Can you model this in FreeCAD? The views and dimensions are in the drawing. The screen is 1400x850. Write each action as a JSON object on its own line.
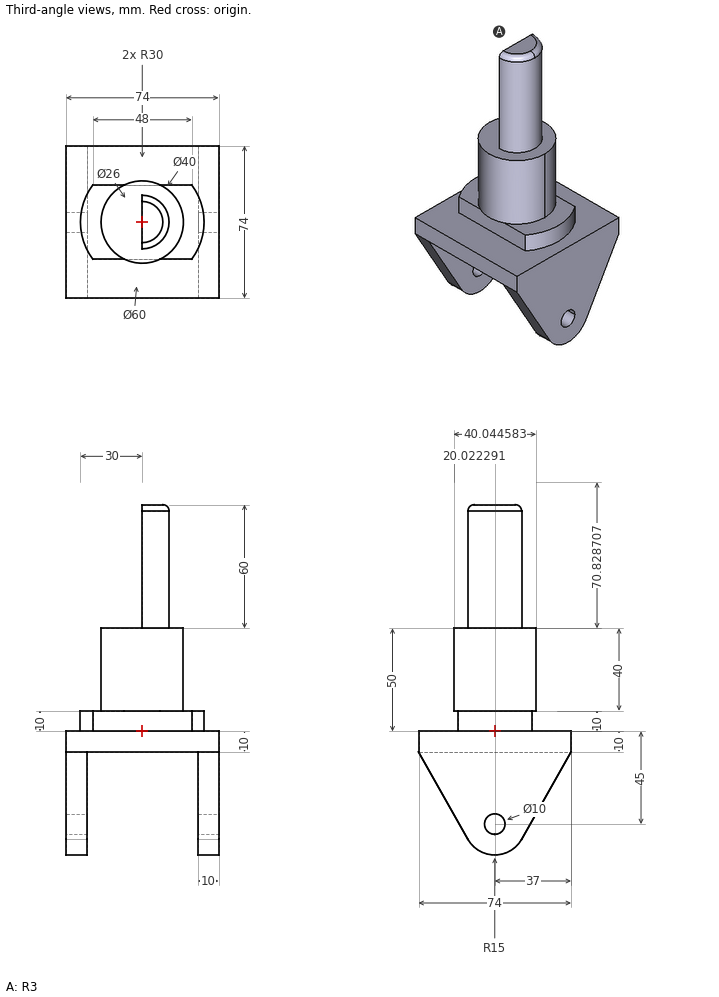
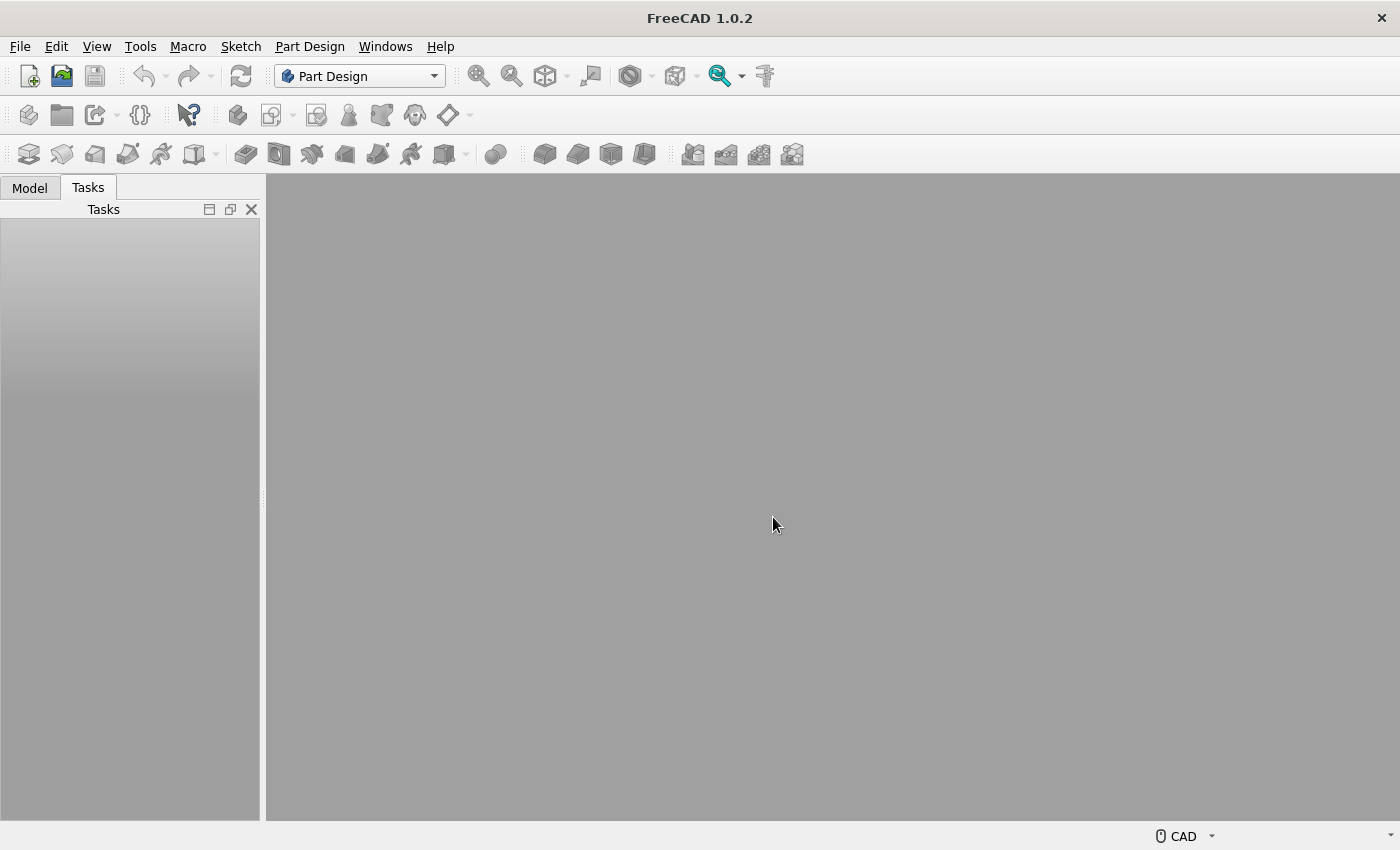
{"action": "key", "text": "ctrl+n"}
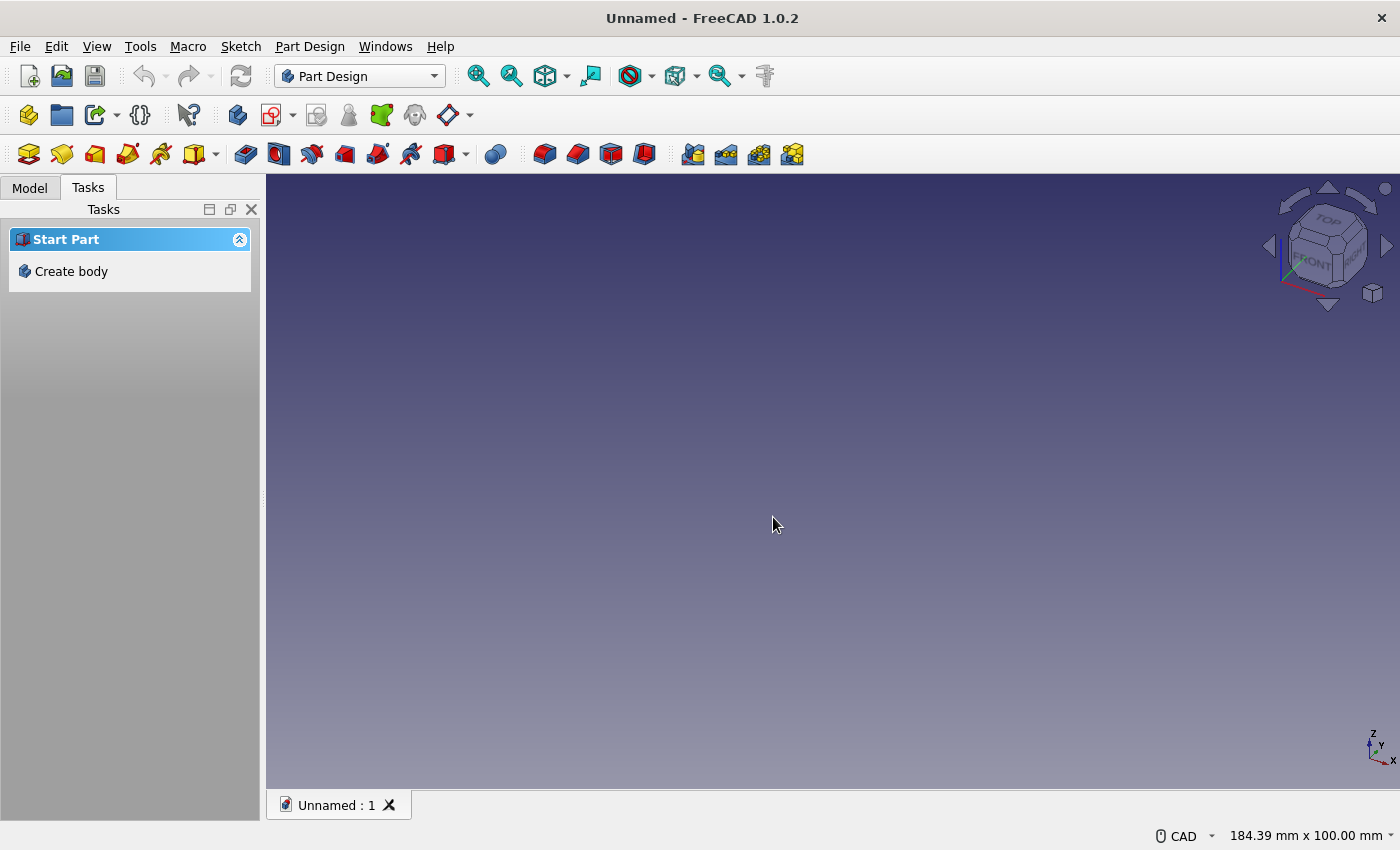
{"action": "left_click", "coordinate": [270, 116]}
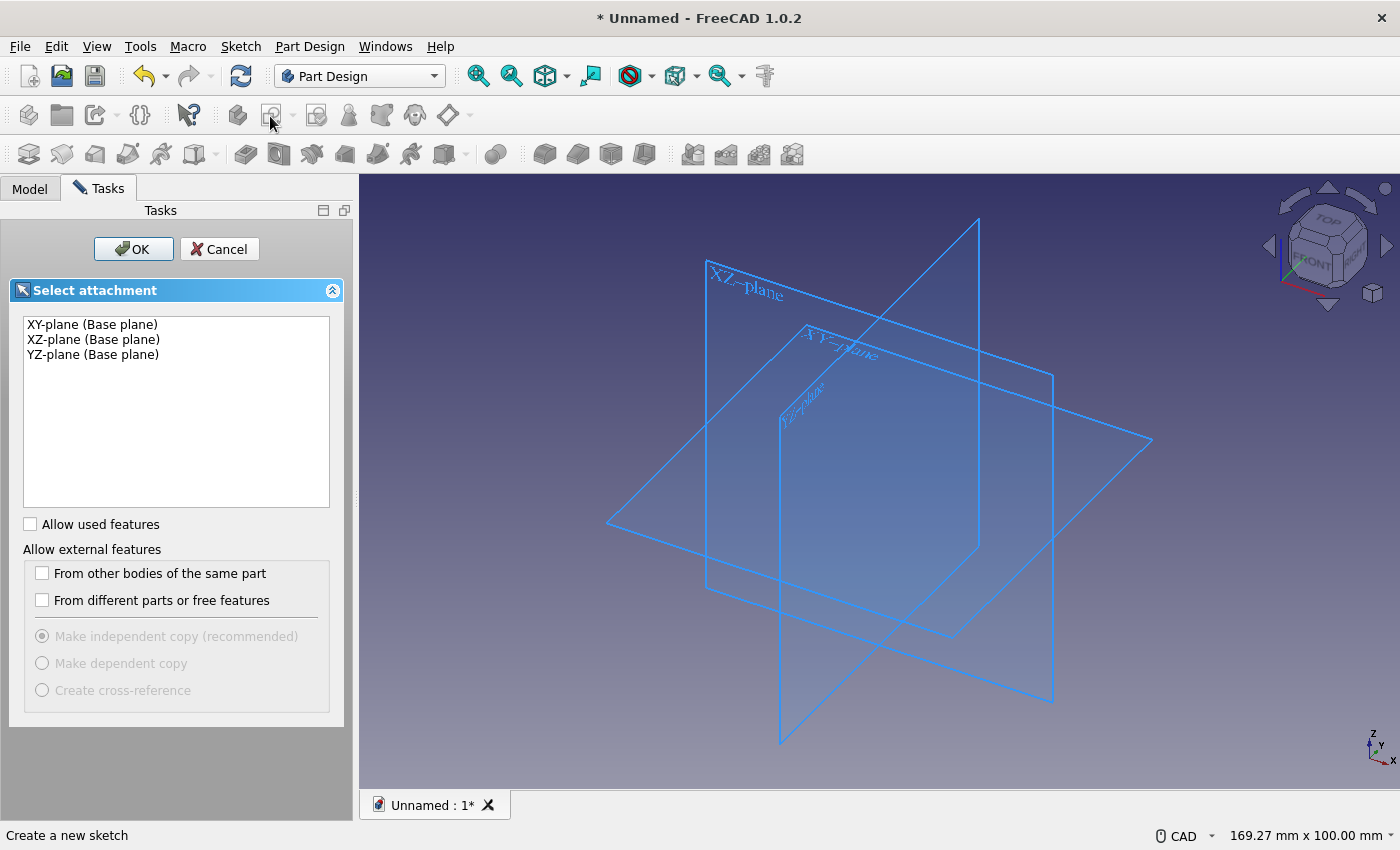
{"action": "left_click", "coordinate": [84, 324]}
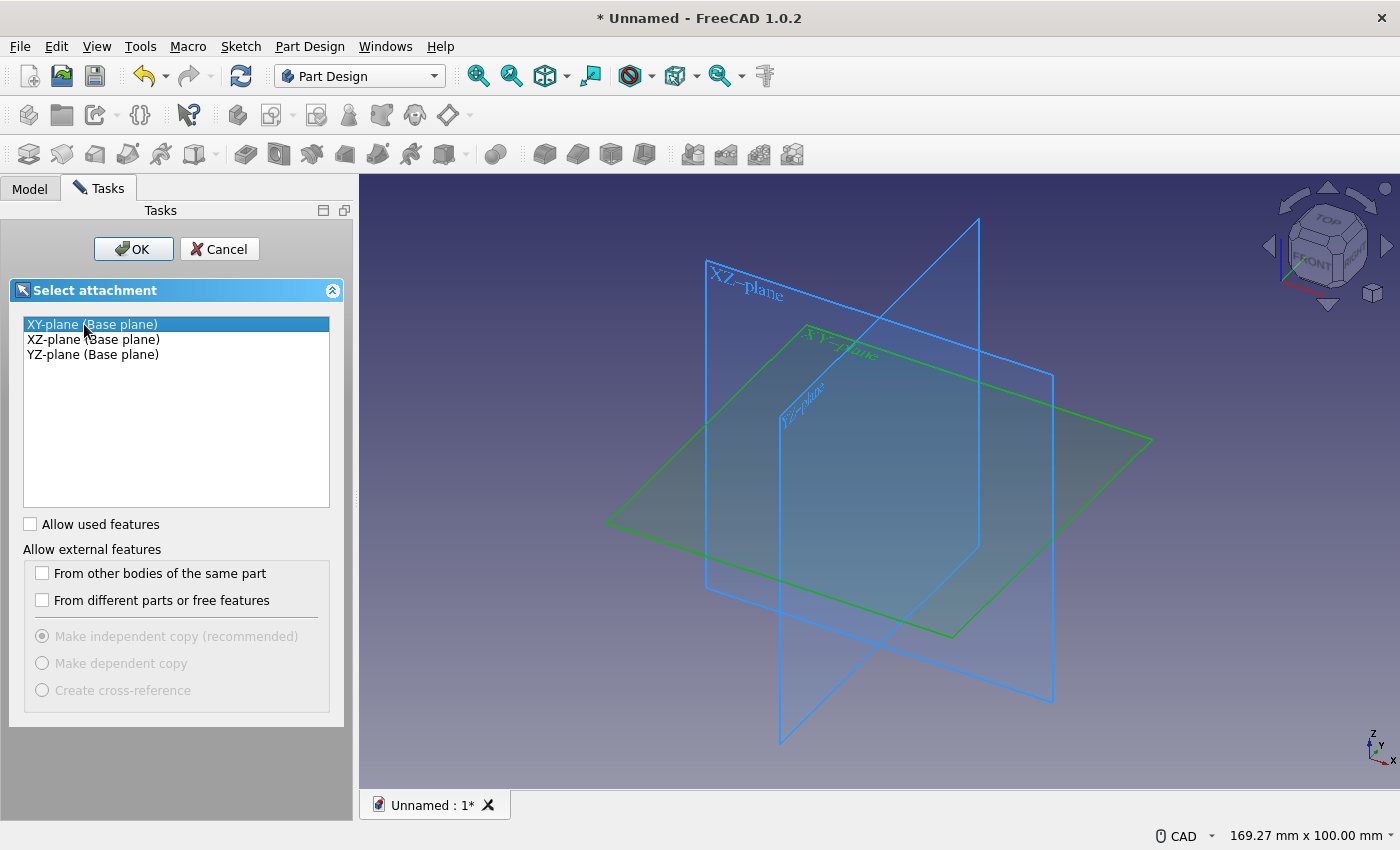
{"action": "left_click", "coordinate": [134, 249]}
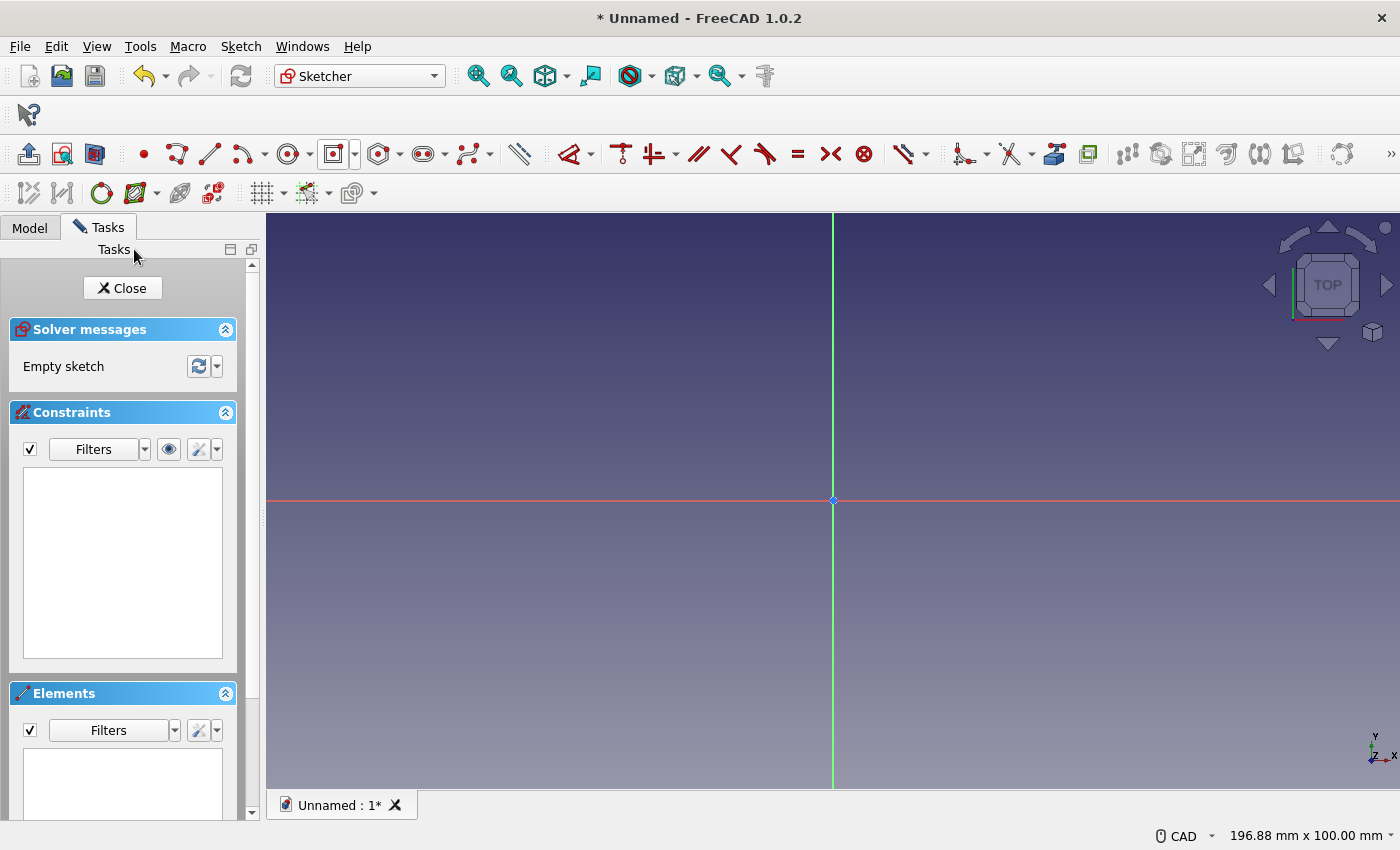
{"action": "key", "text": "g c"}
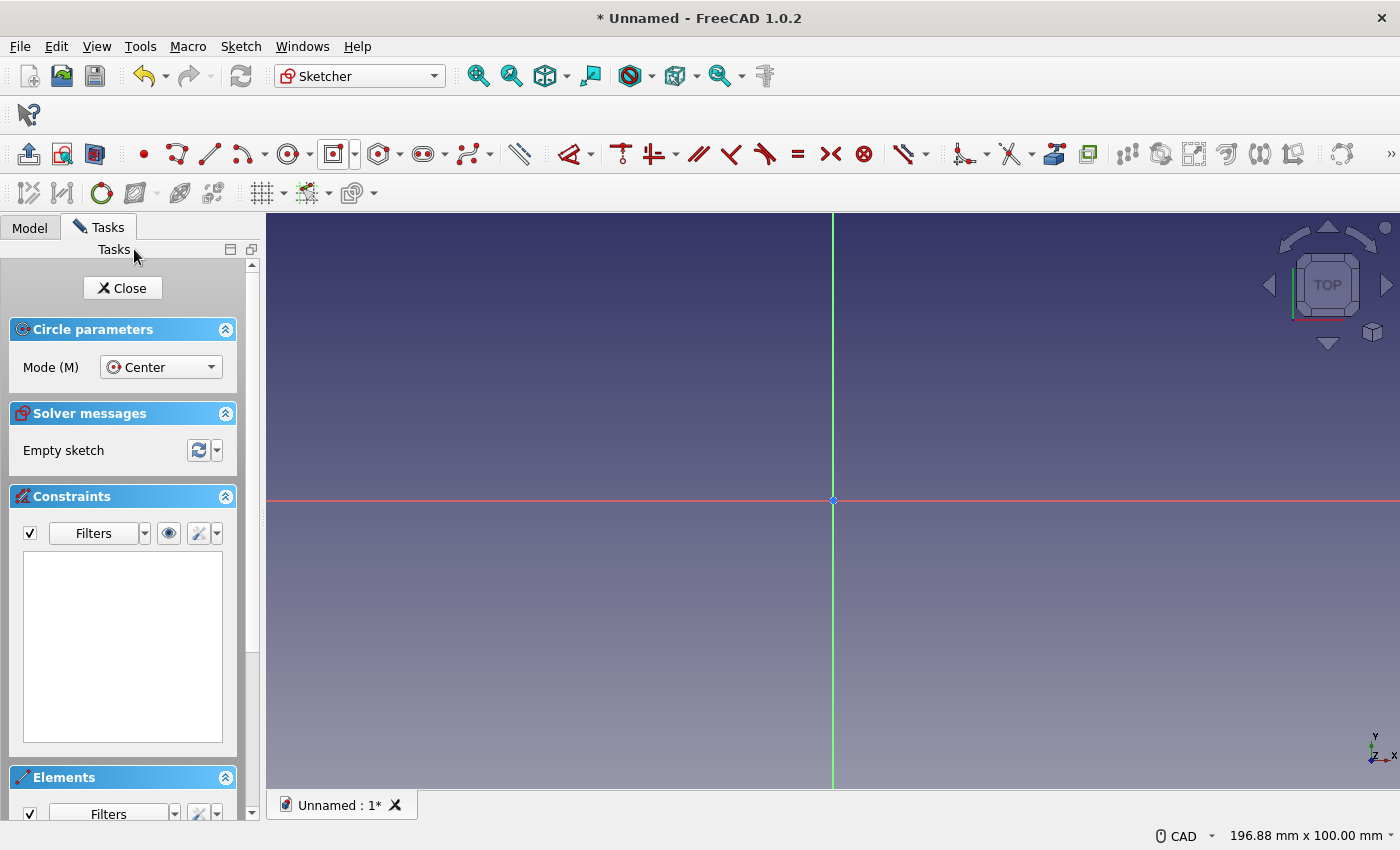
{"action": "left_click", "coordinate": [833, 501]}
{"action": "mouse_move", "coordinate": [955, 379]}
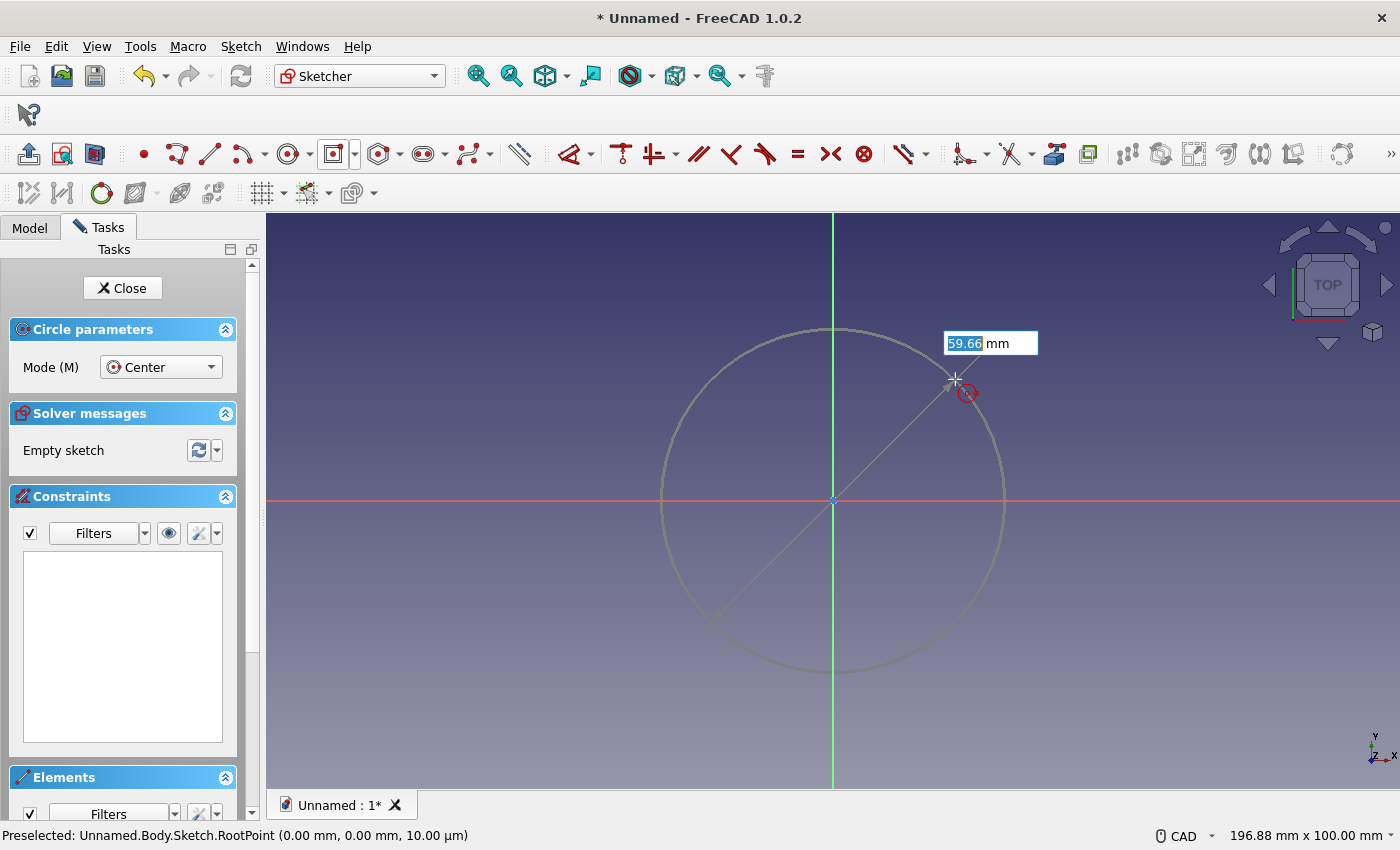
{"action": "type", "text": "60"}
{"action": "key", "text": "Return"}
{"action": "key", "text": "Escape"}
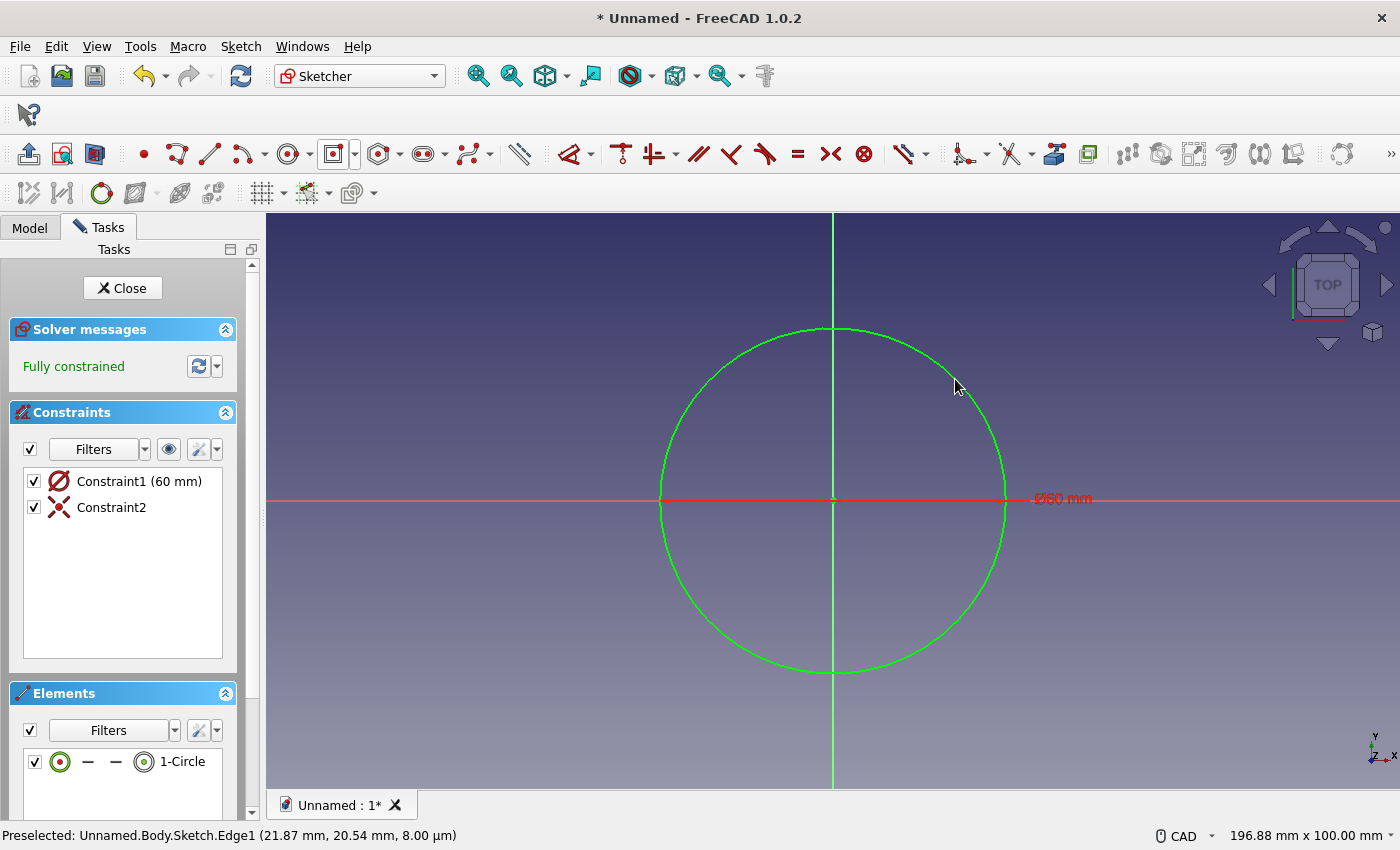
{"action": "left_click", "coordinate": [123, 288]}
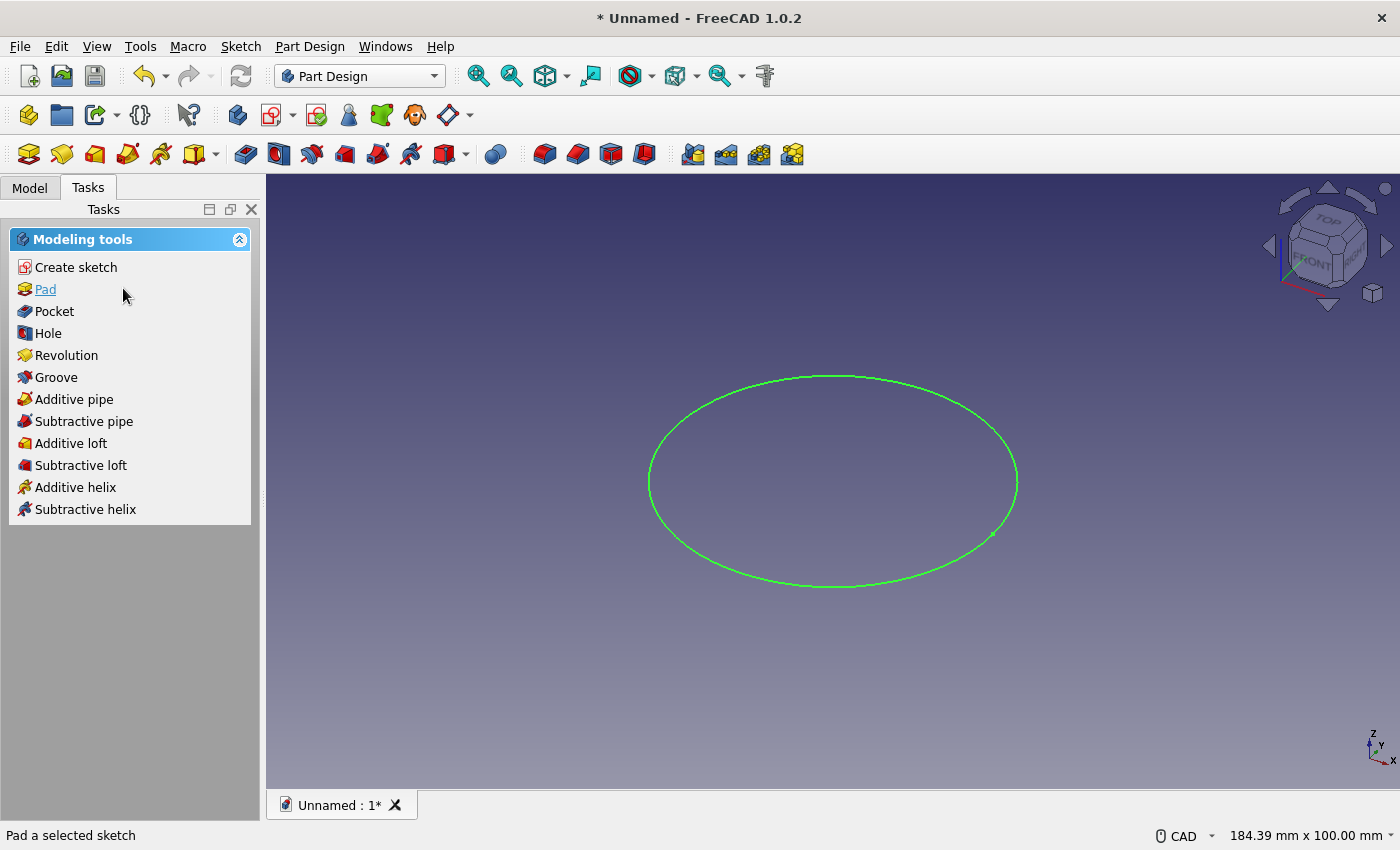
{"action": "left_click", "coordinate": [29, 154]}